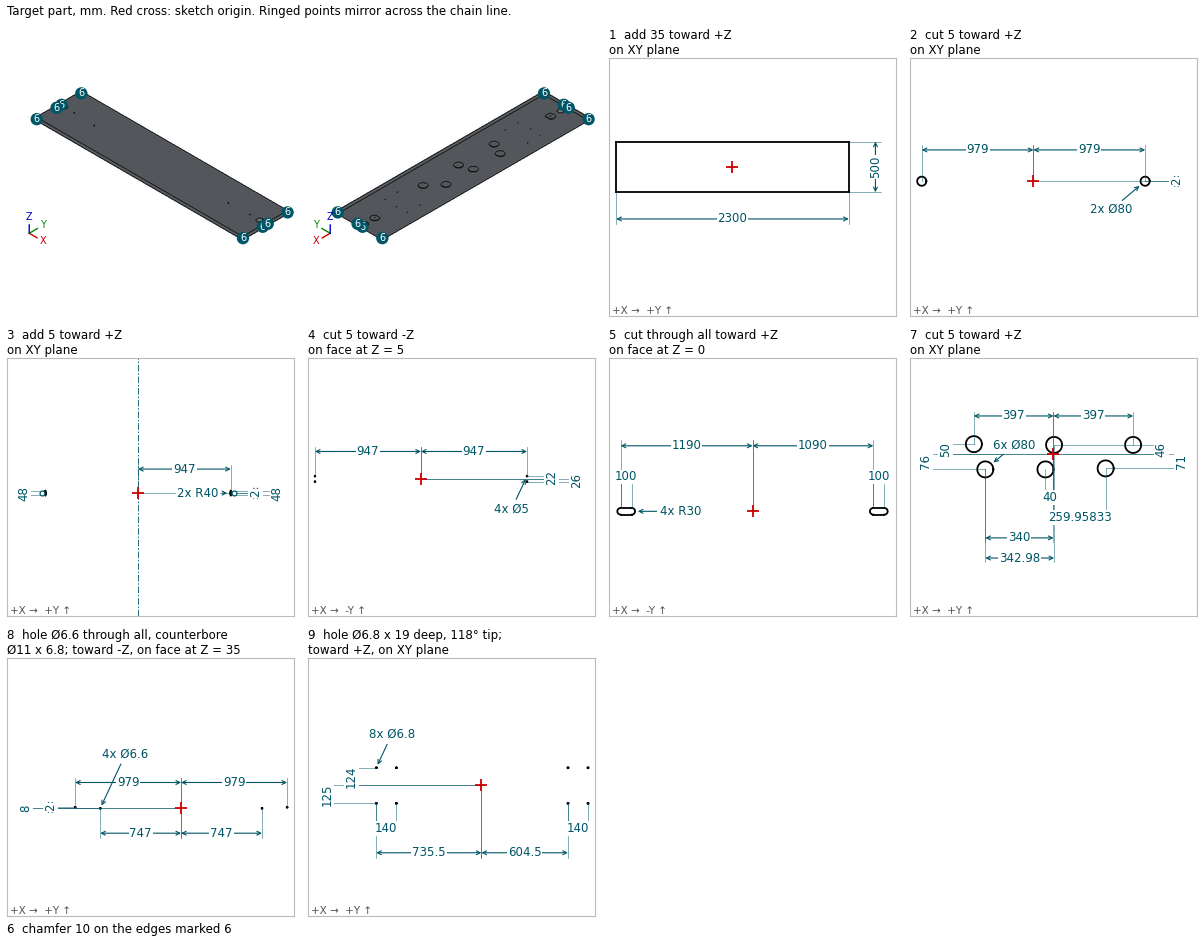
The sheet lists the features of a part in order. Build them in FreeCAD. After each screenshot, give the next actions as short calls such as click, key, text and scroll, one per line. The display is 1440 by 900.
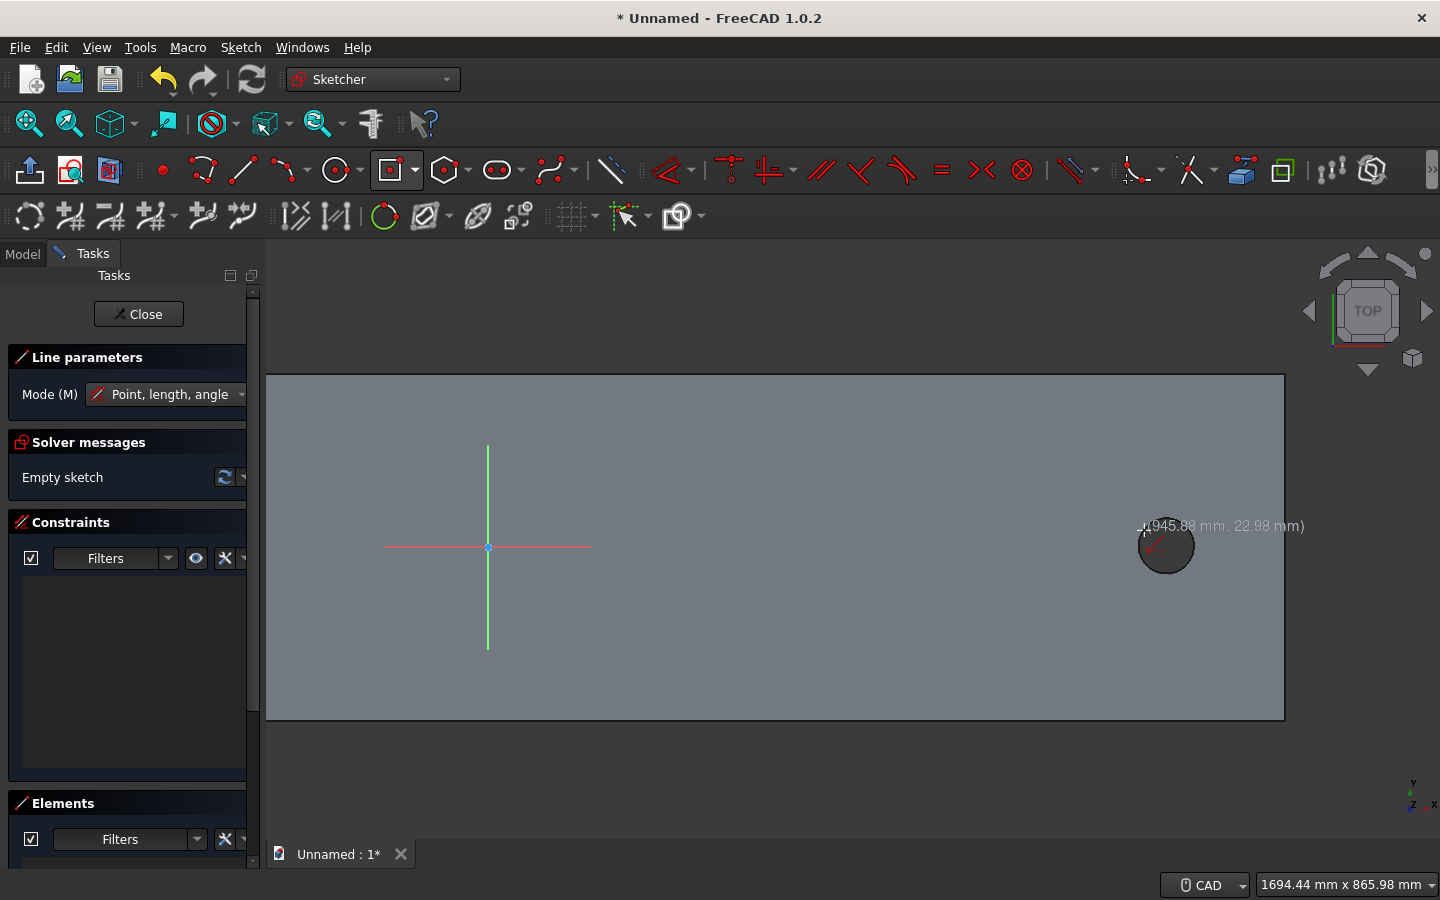
click(1144, 529)
click(1144, 563)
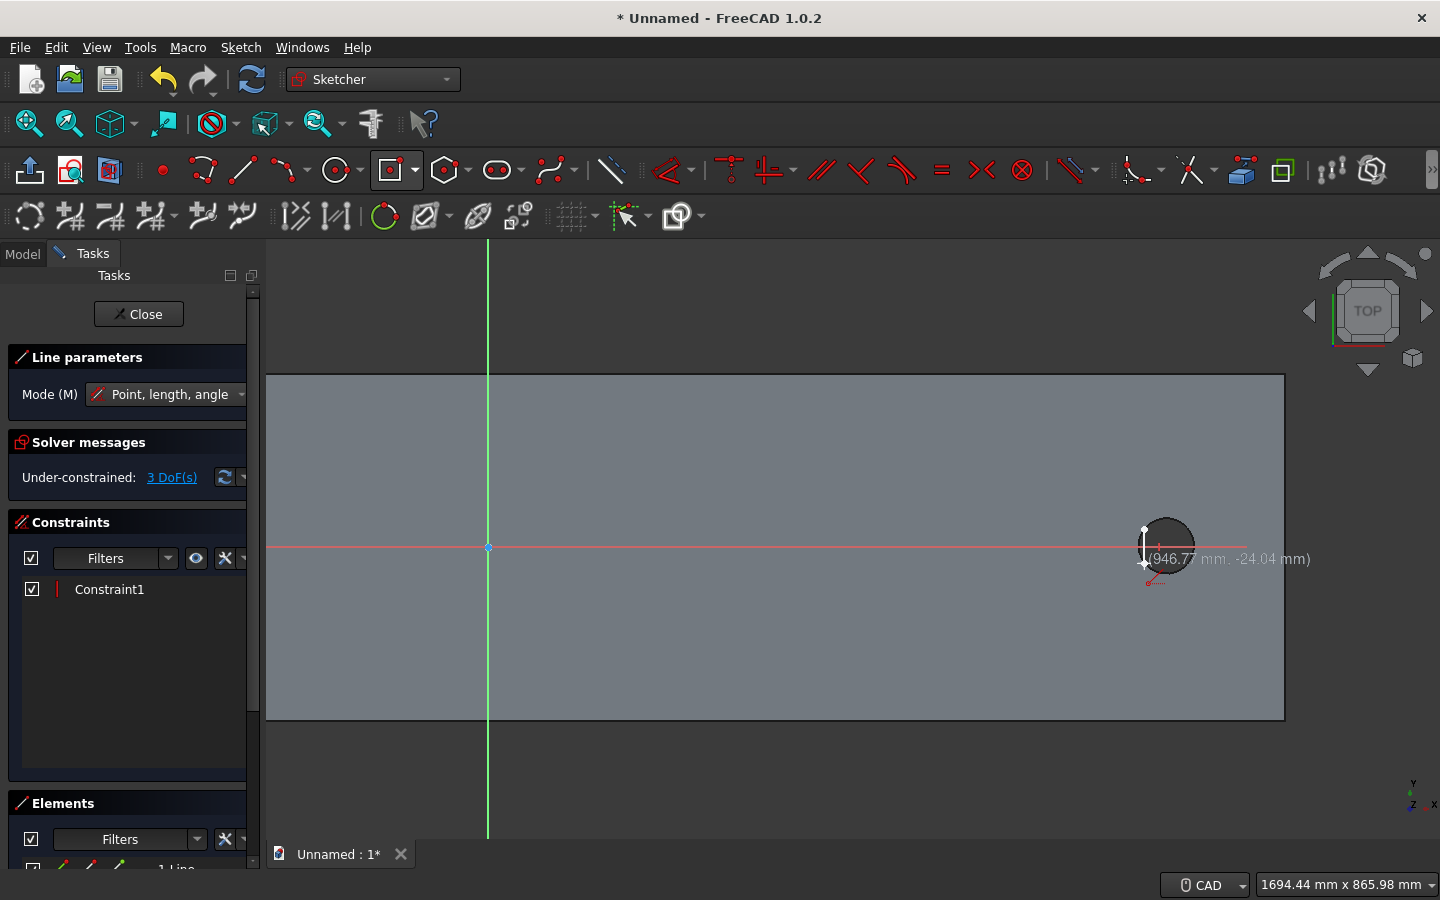
click(284, 170)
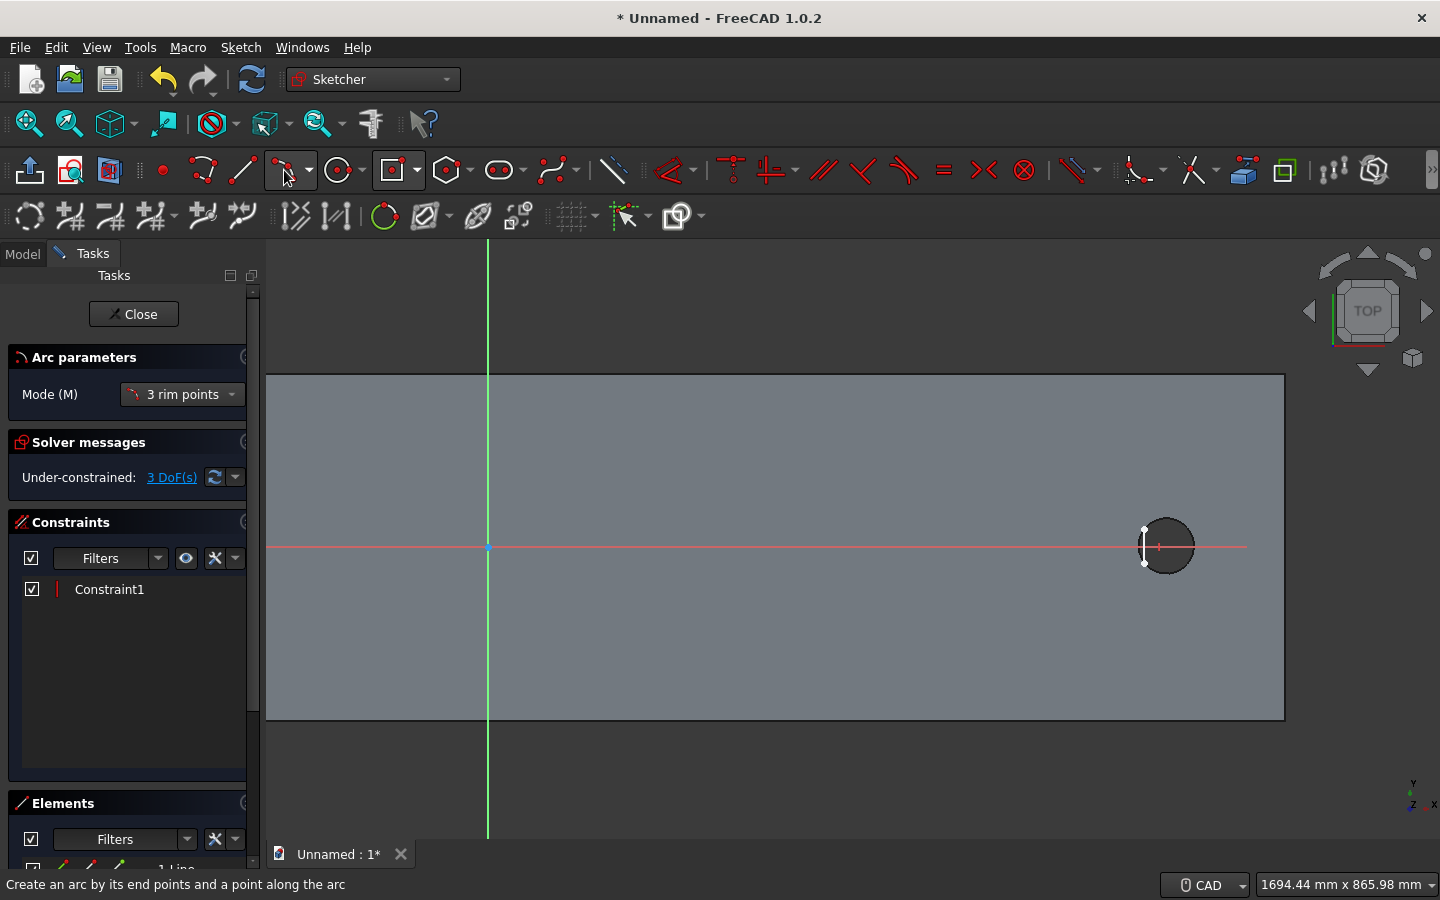
click(1144, 564)
click(1144, 530)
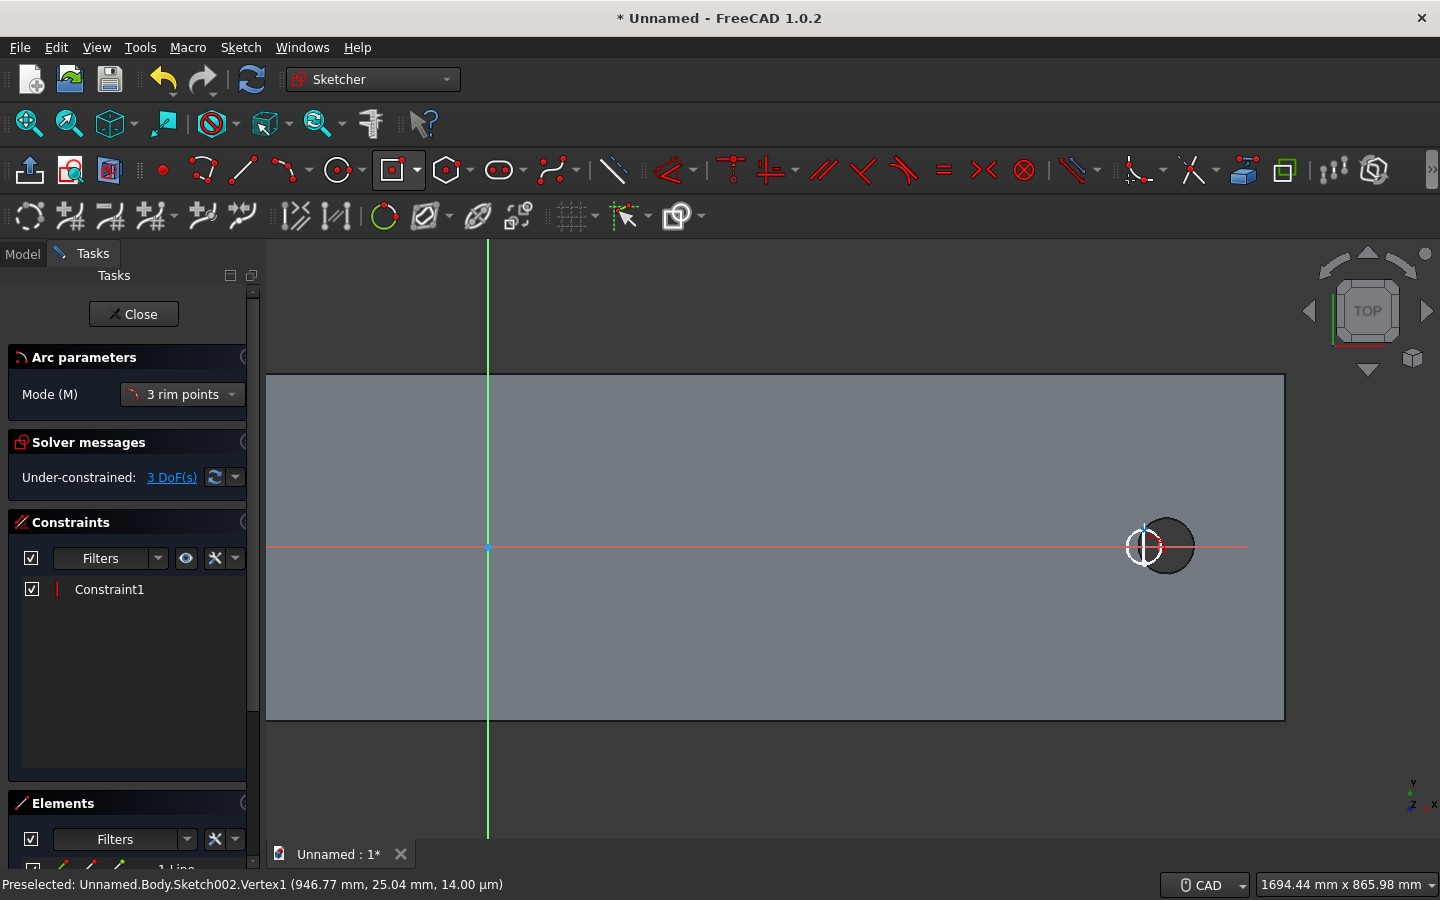
scroll(1139, 542, up, 6)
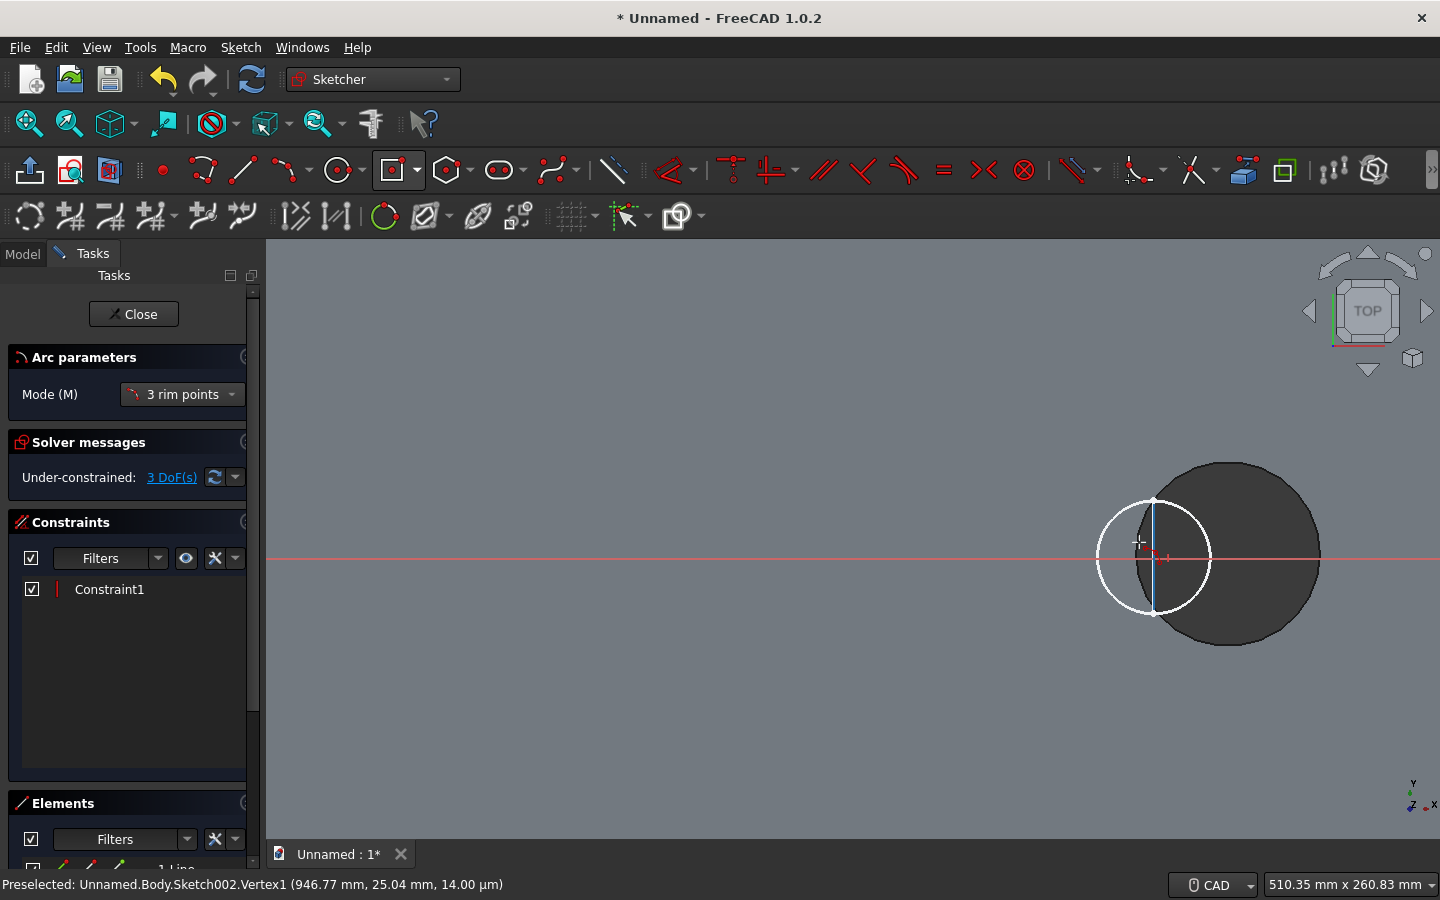
click(1137, 542)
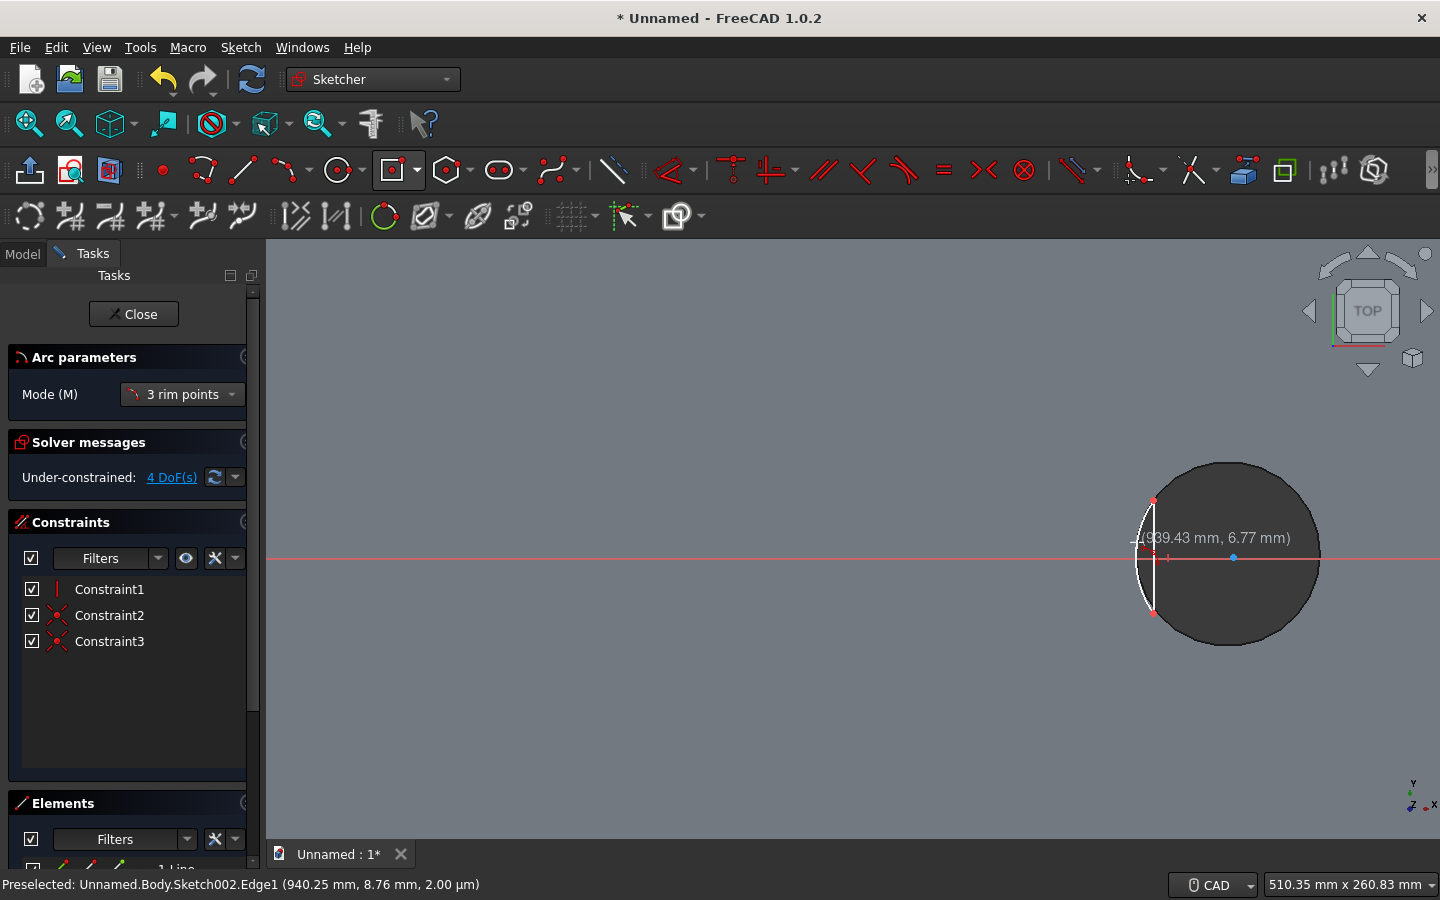
click(244, 170)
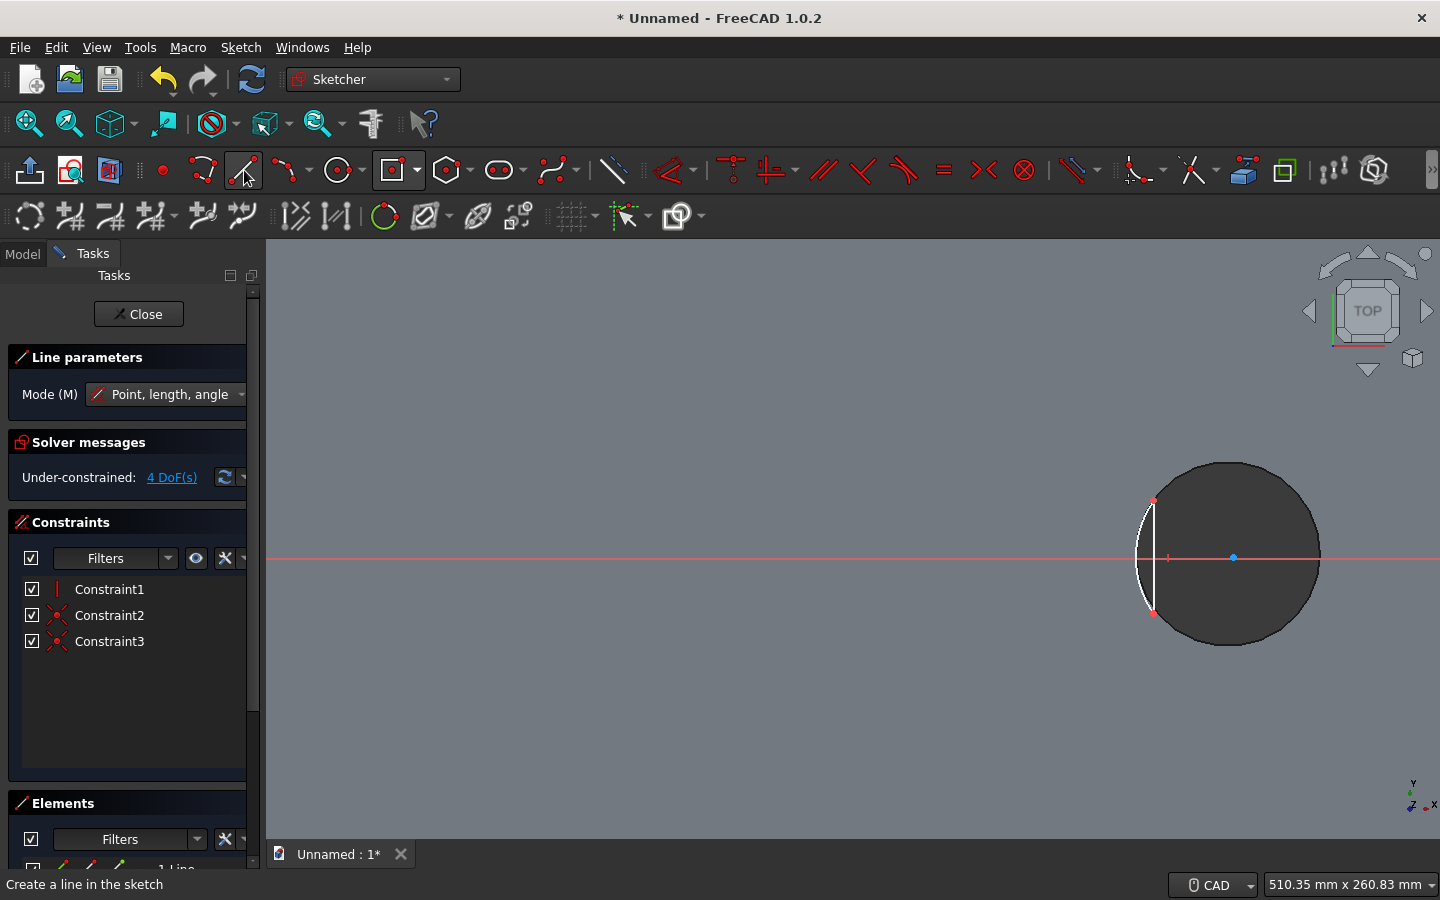
scroll(1143, 536, down, 9)